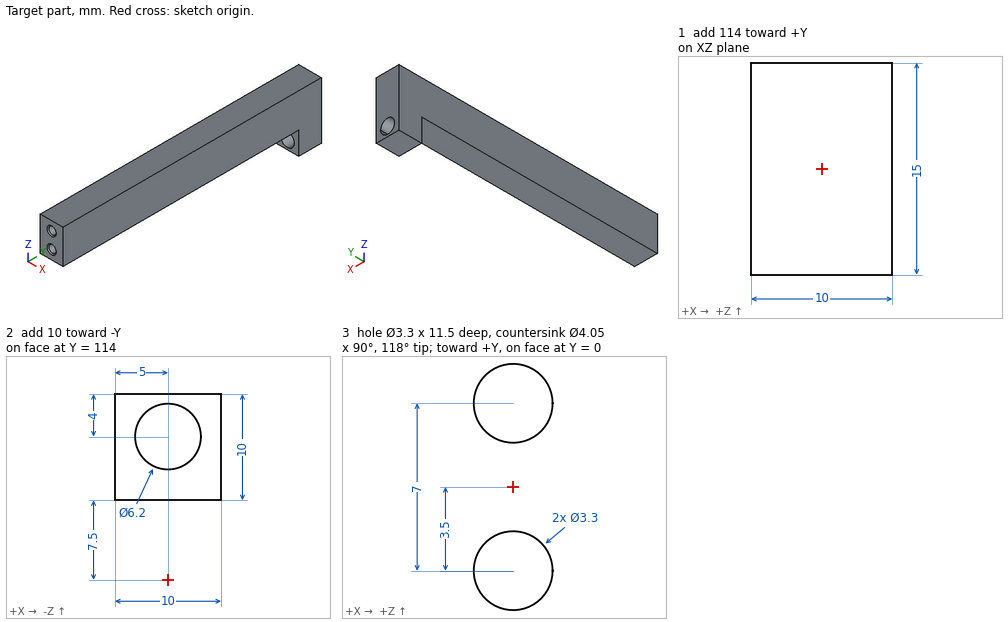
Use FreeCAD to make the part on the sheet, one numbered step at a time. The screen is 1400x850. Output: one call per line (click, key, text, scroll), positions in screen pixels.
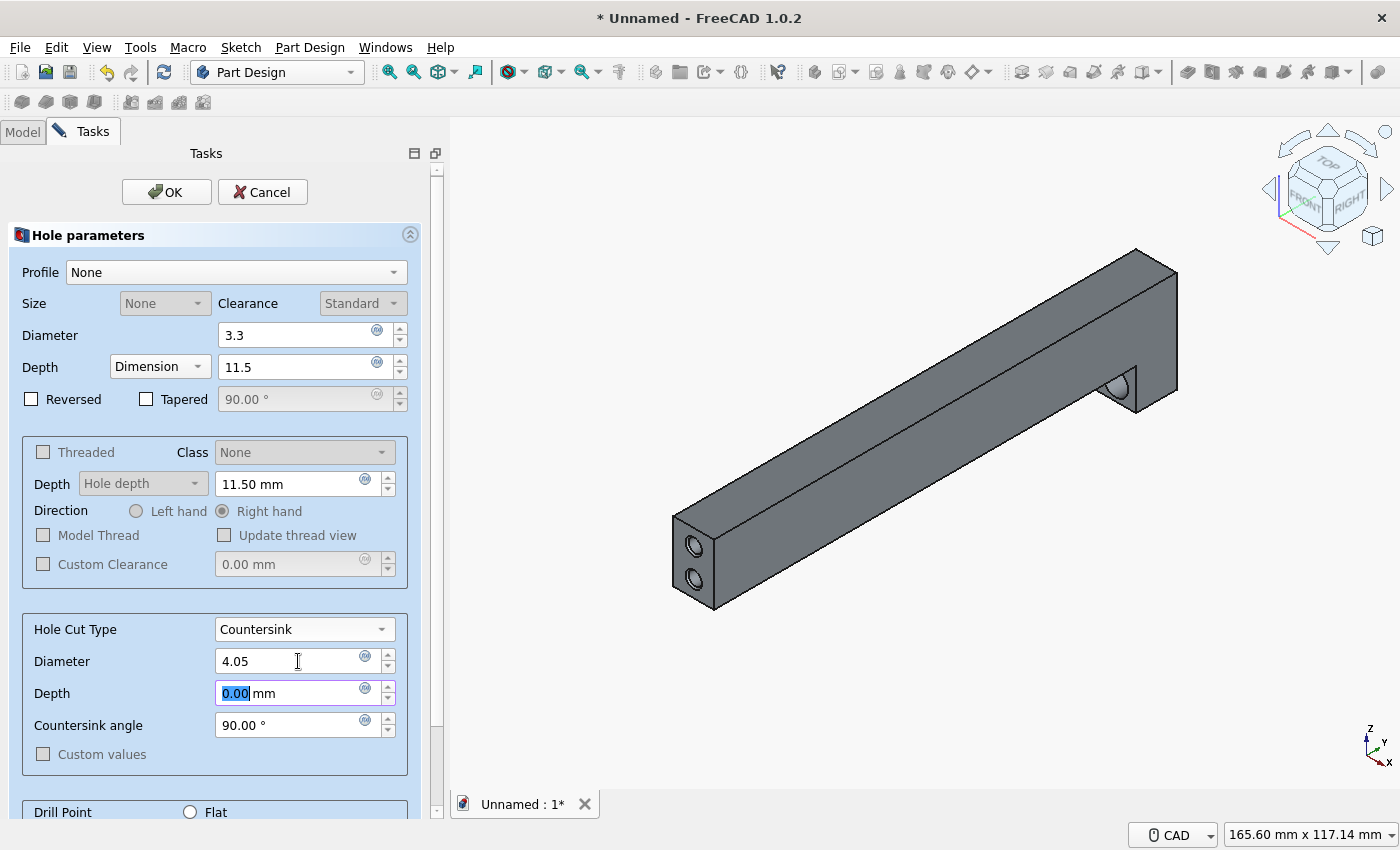
click(167, 192)